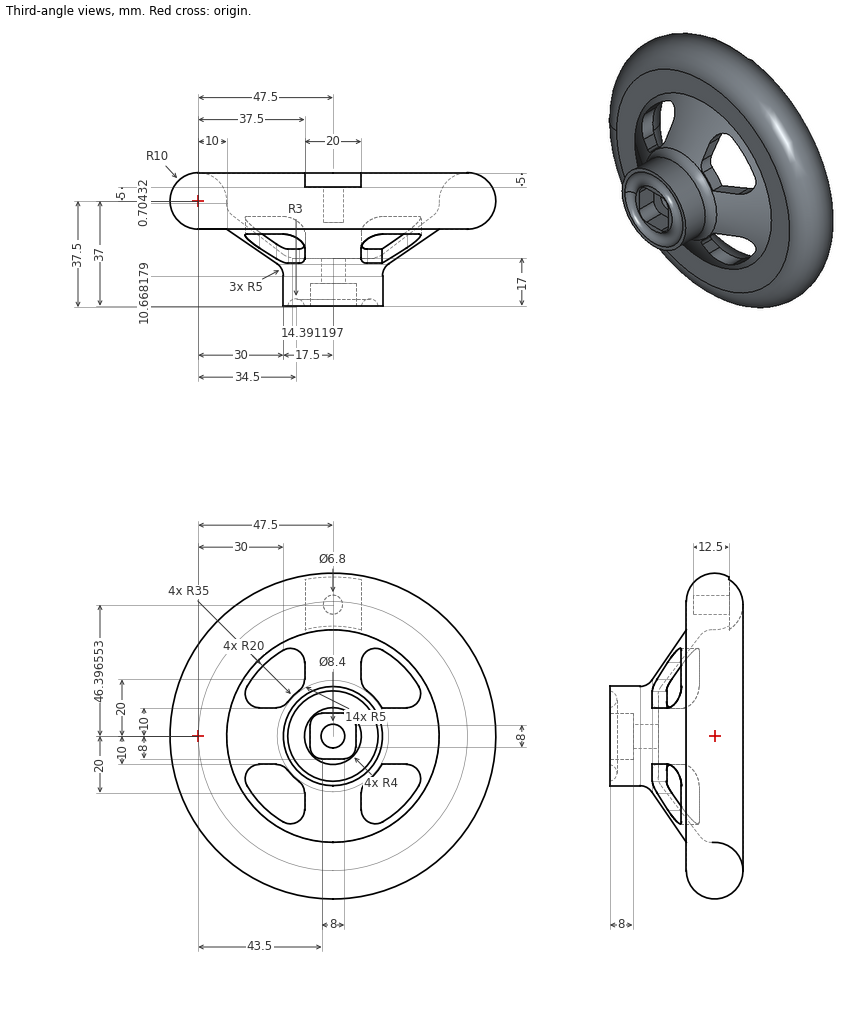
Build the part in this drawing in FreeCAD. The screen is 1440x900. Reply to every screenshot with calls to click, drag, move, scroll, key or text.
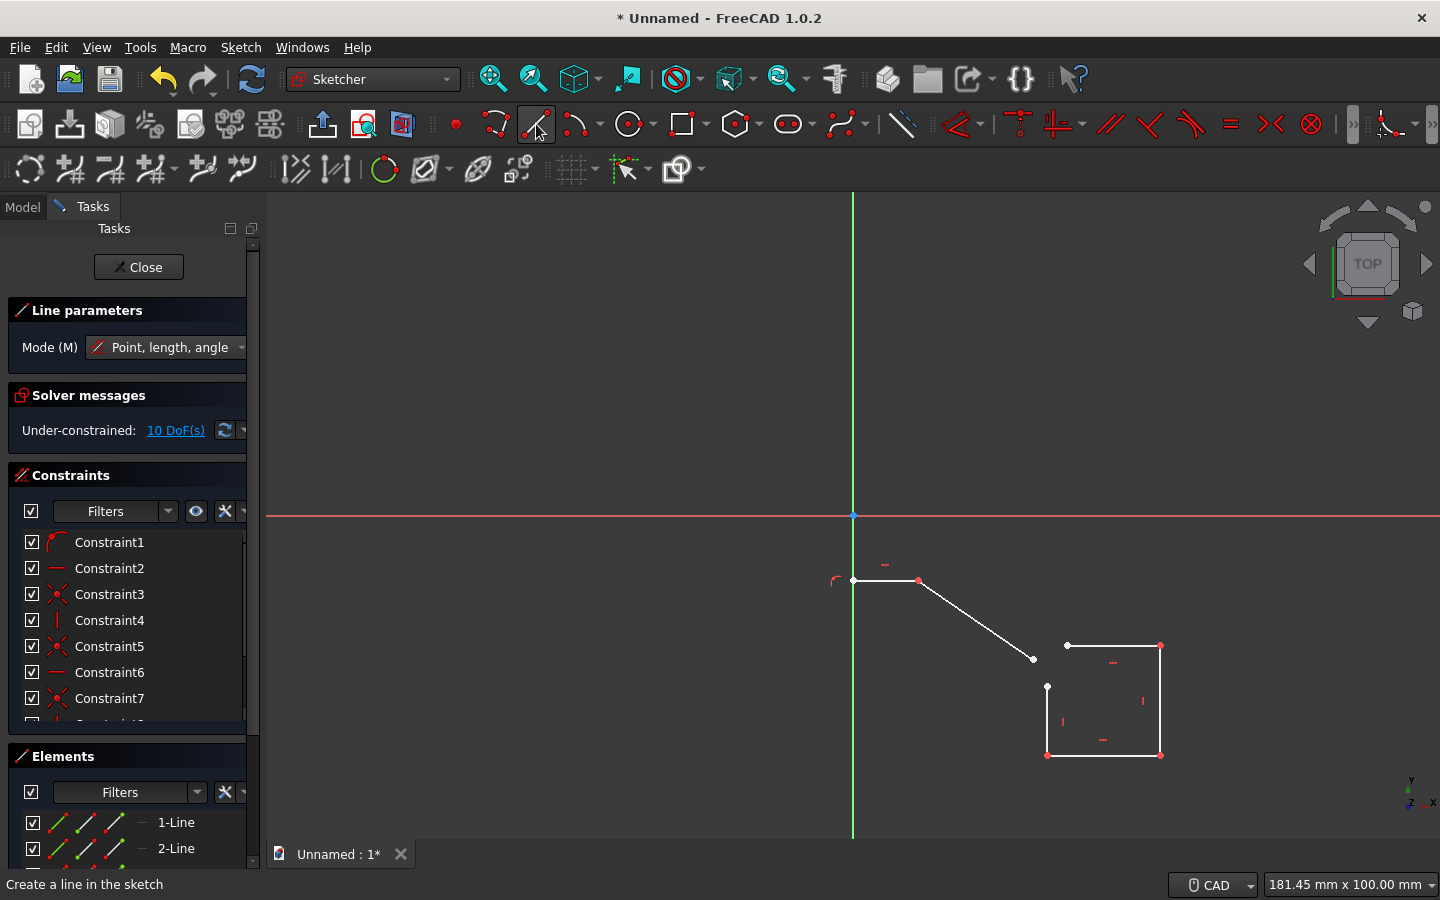
click(1048, 638)
click(930, 548)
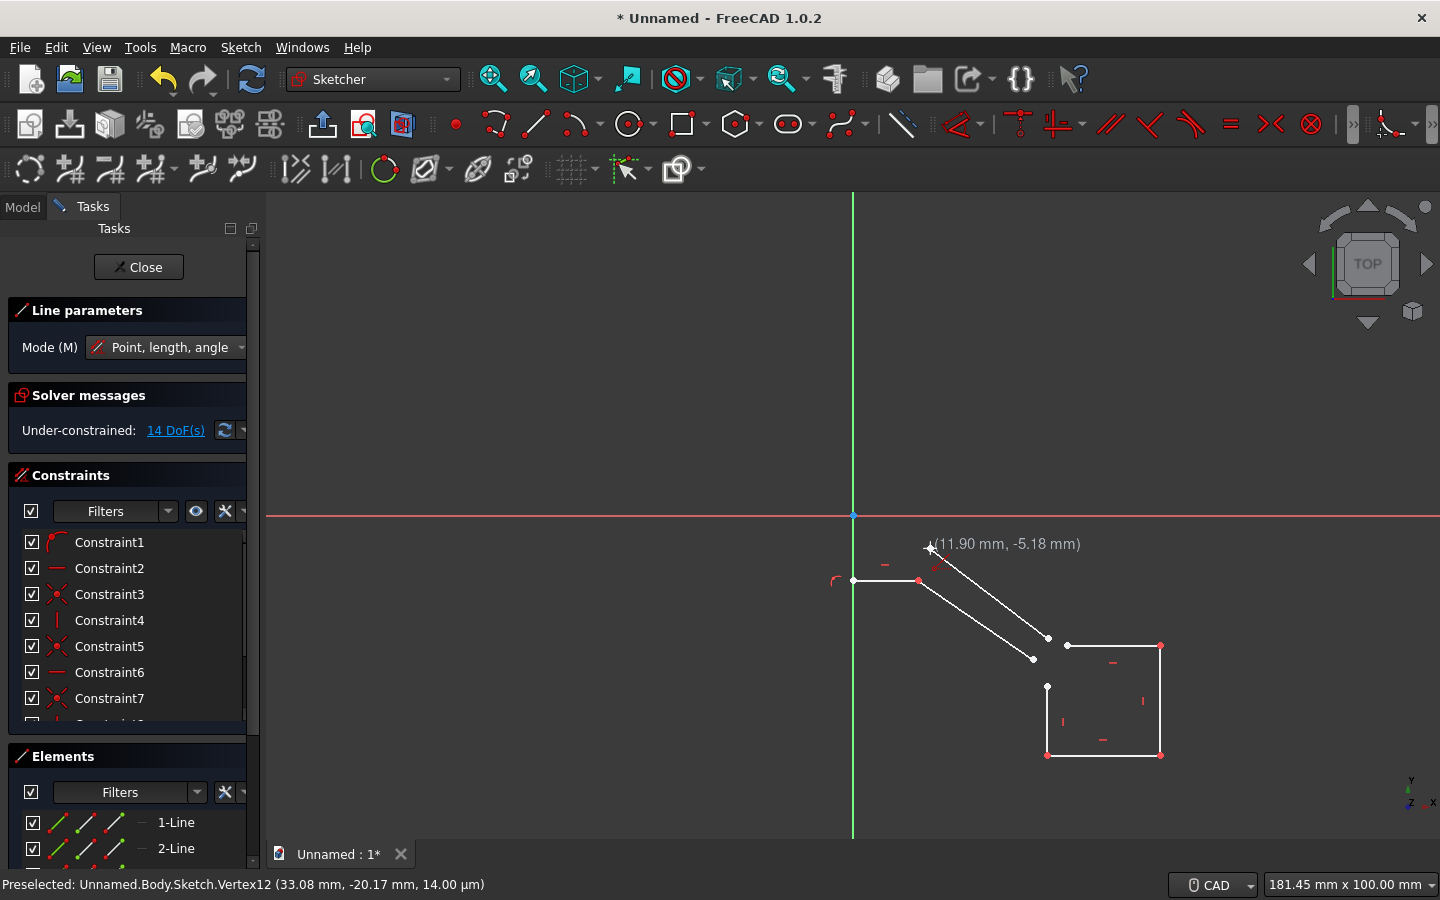
key(g)
key(3)
key(a)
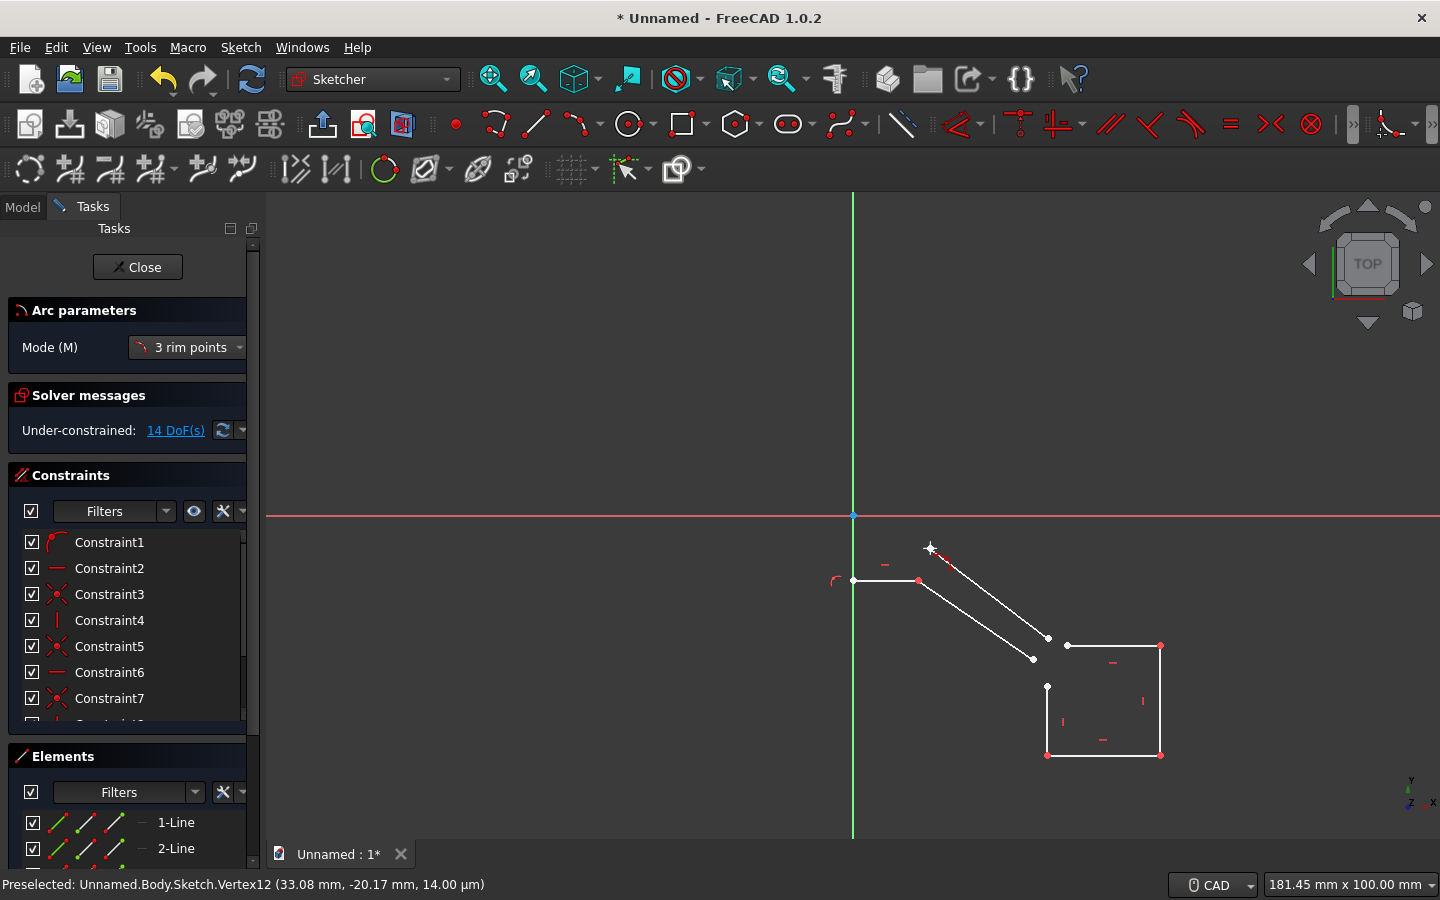
click(1033, 660)
click(1047, 687)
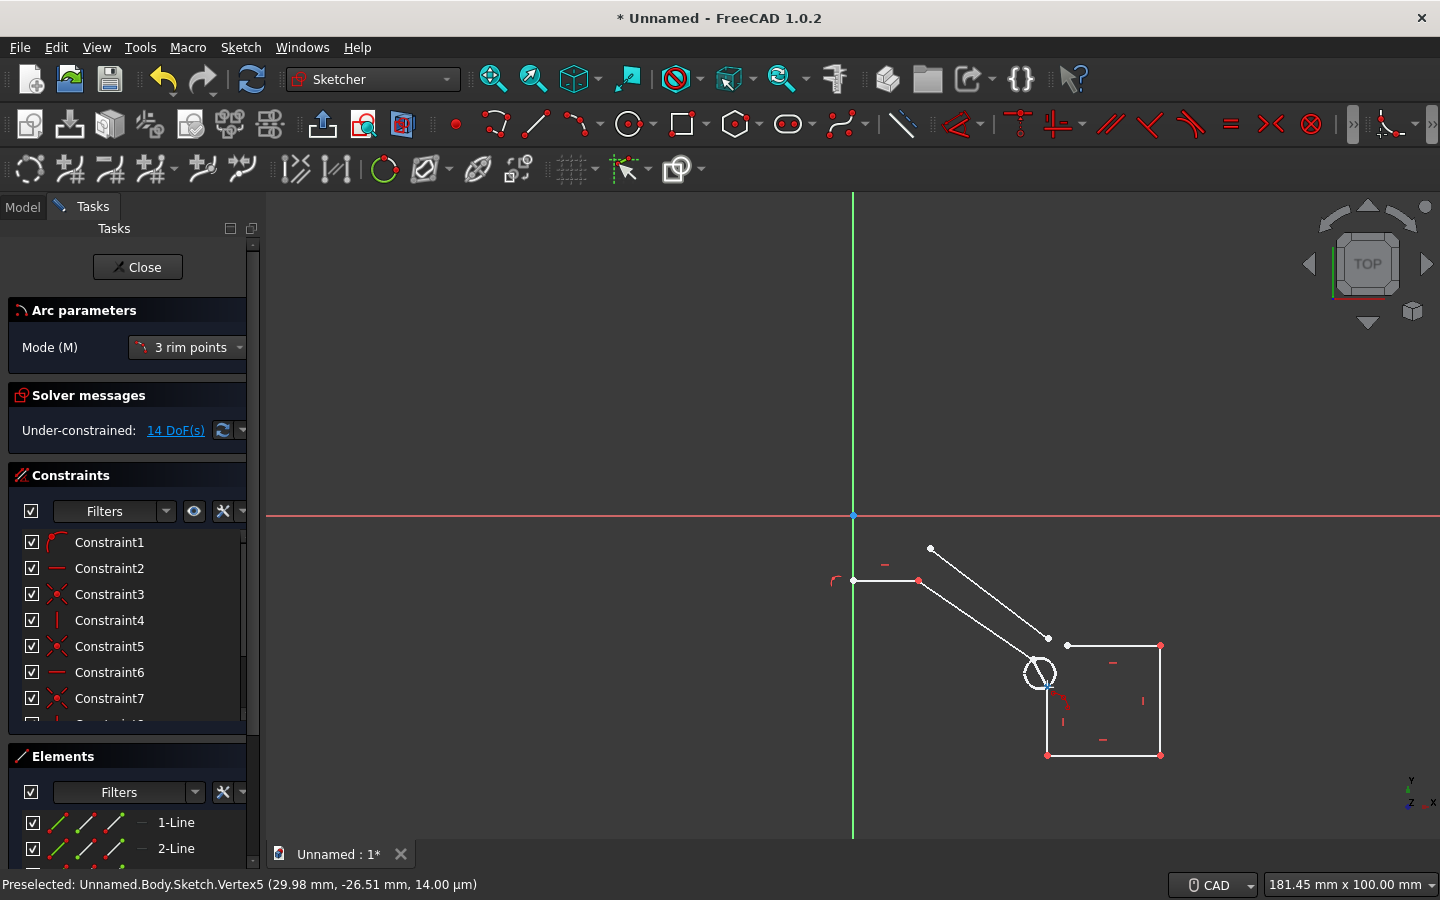
scroll(1043, 671, up, 8)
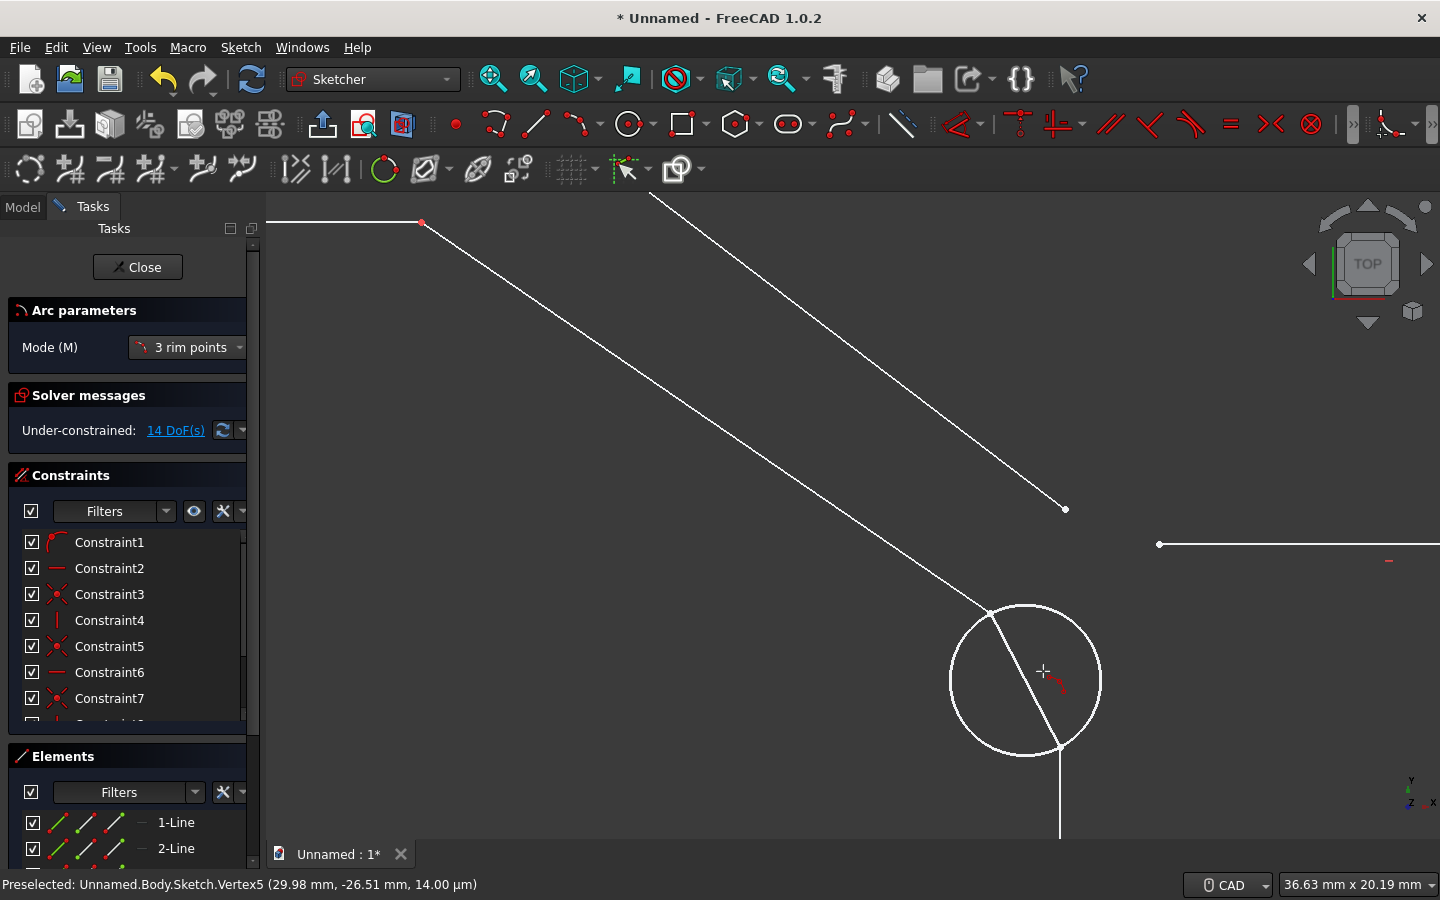
click(1042, 667)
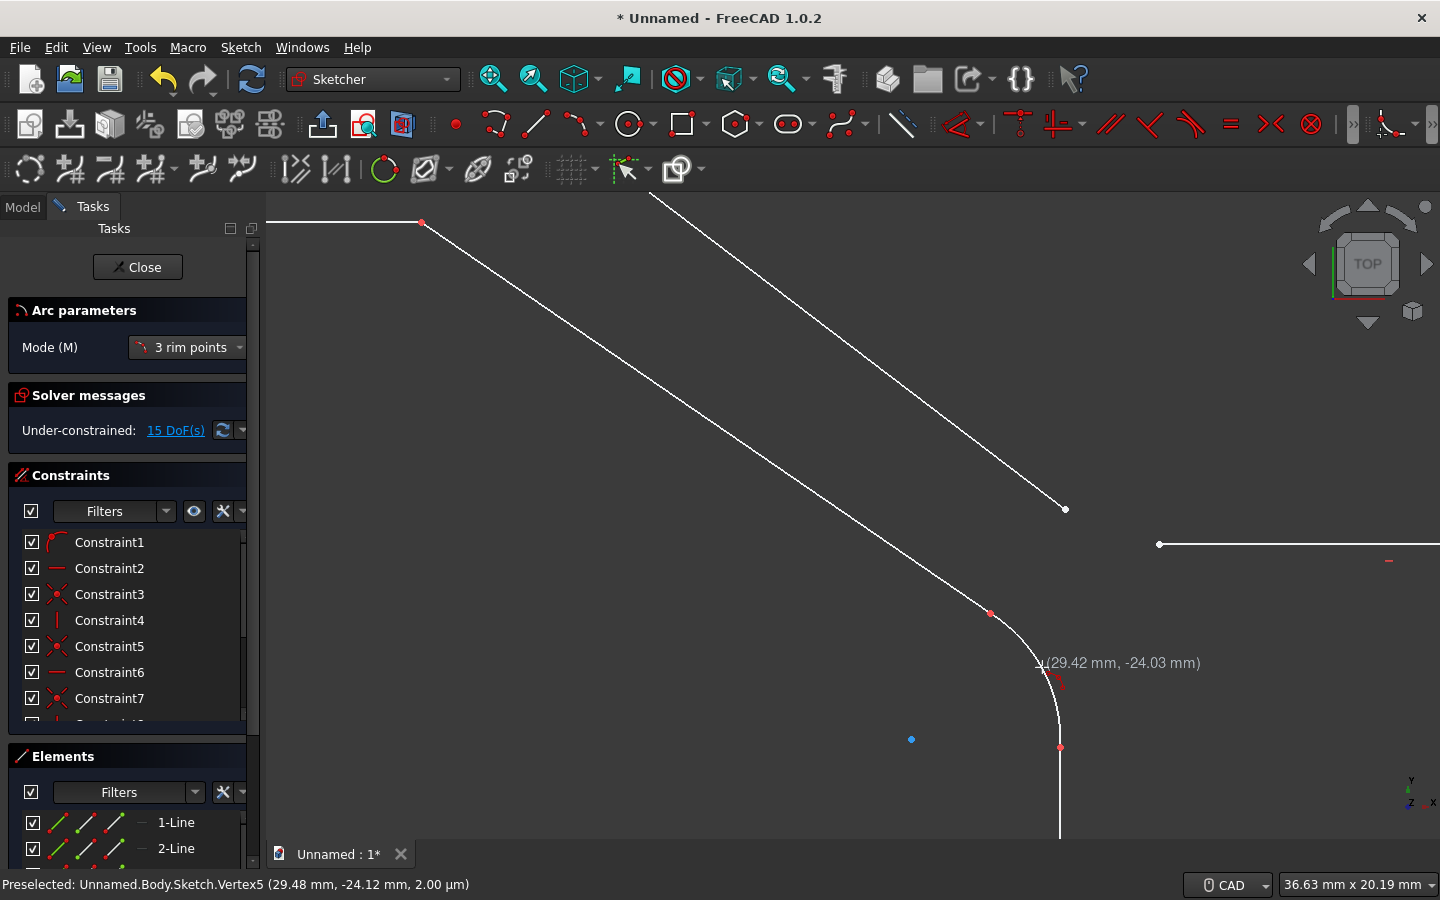
scroll(793, 623, down, 8)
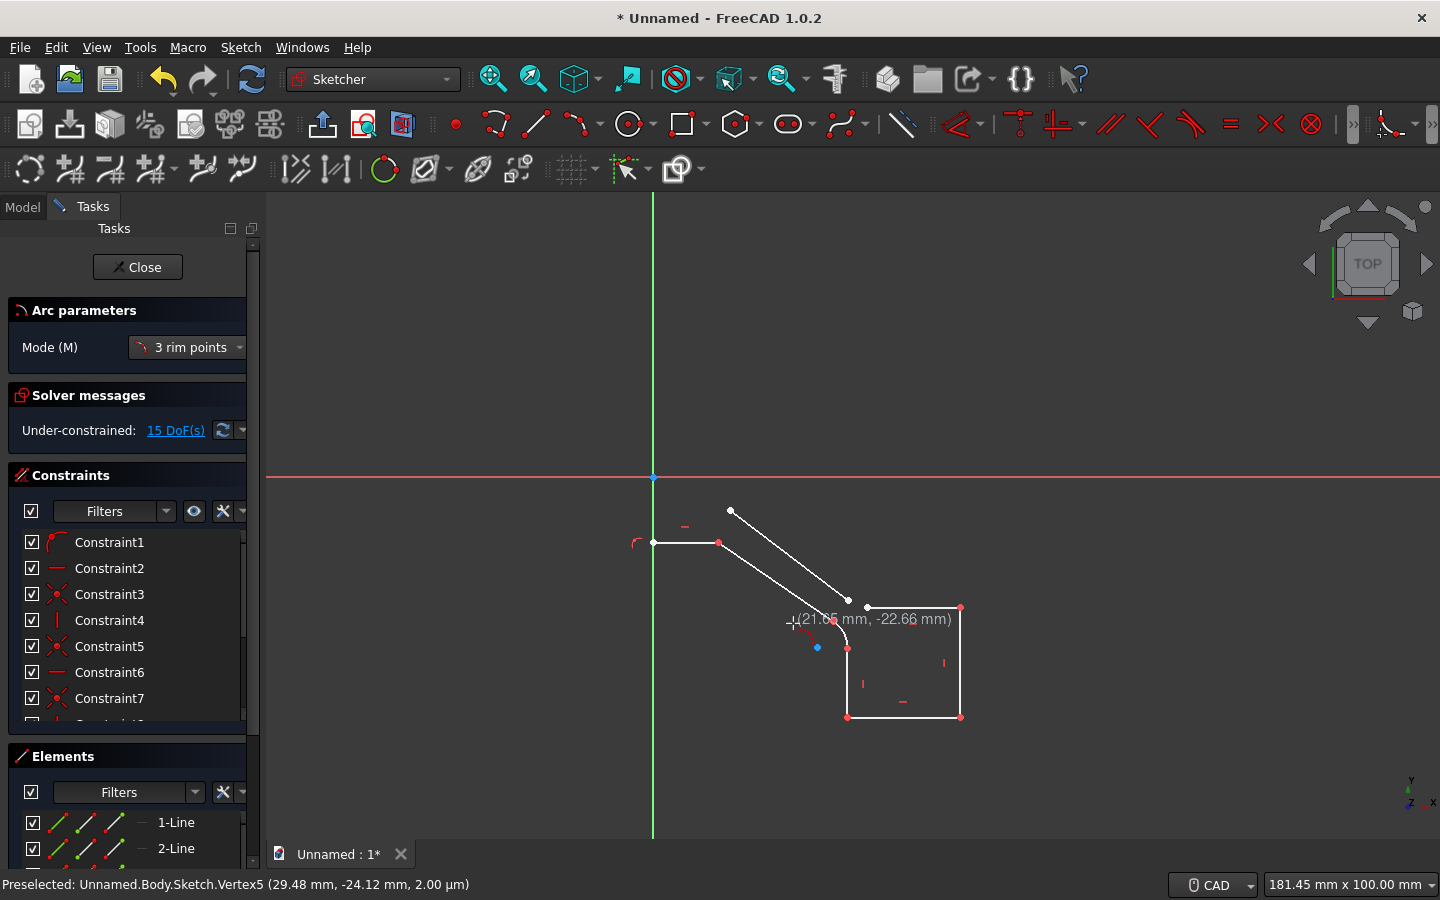
click(867, 608)
click(848, 601)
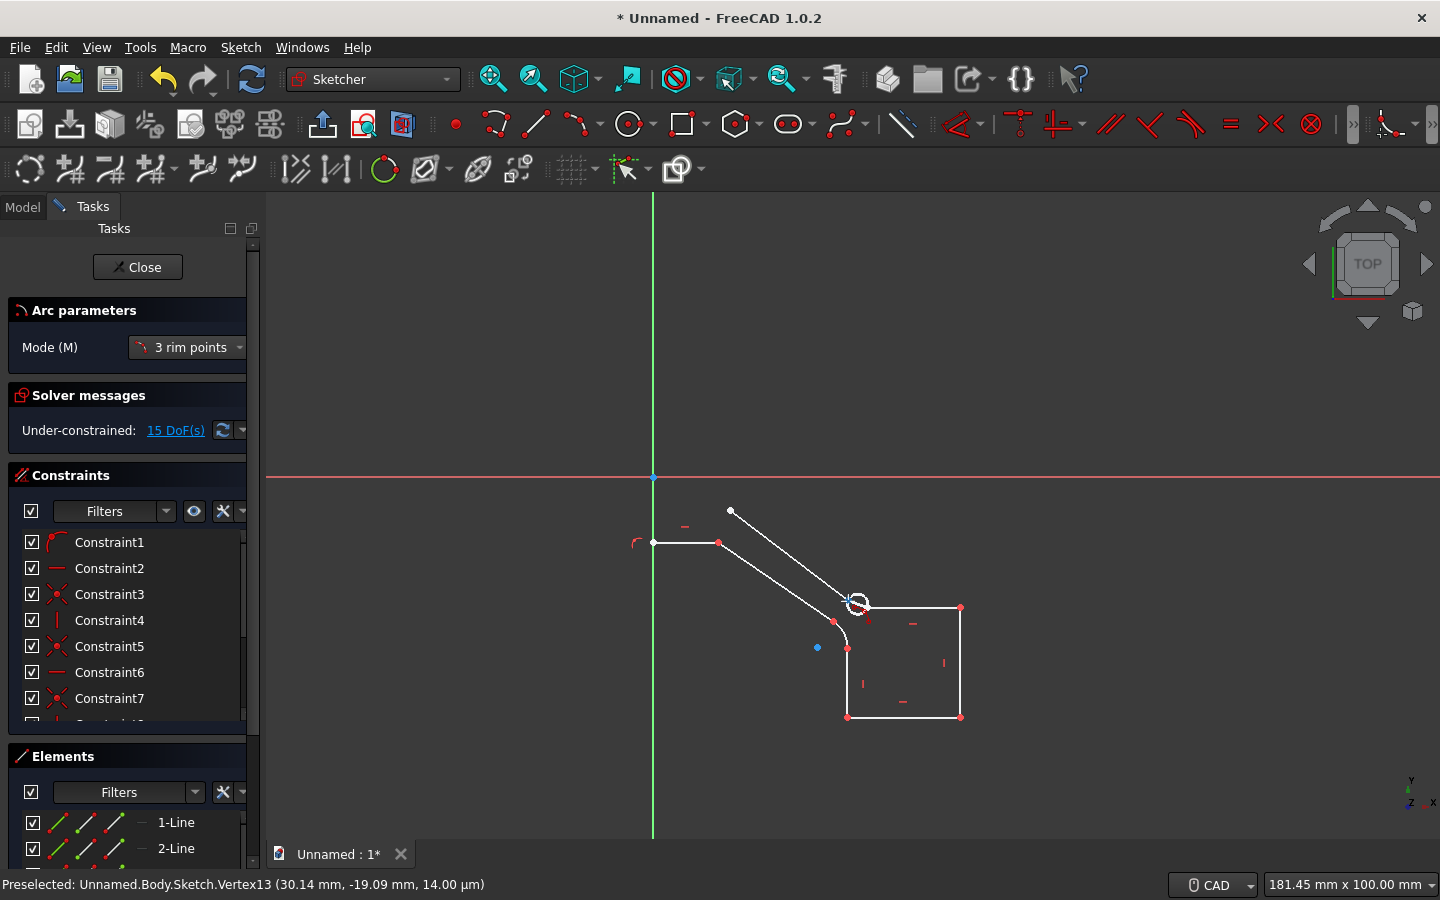
scroll(857, 605, up, 12)